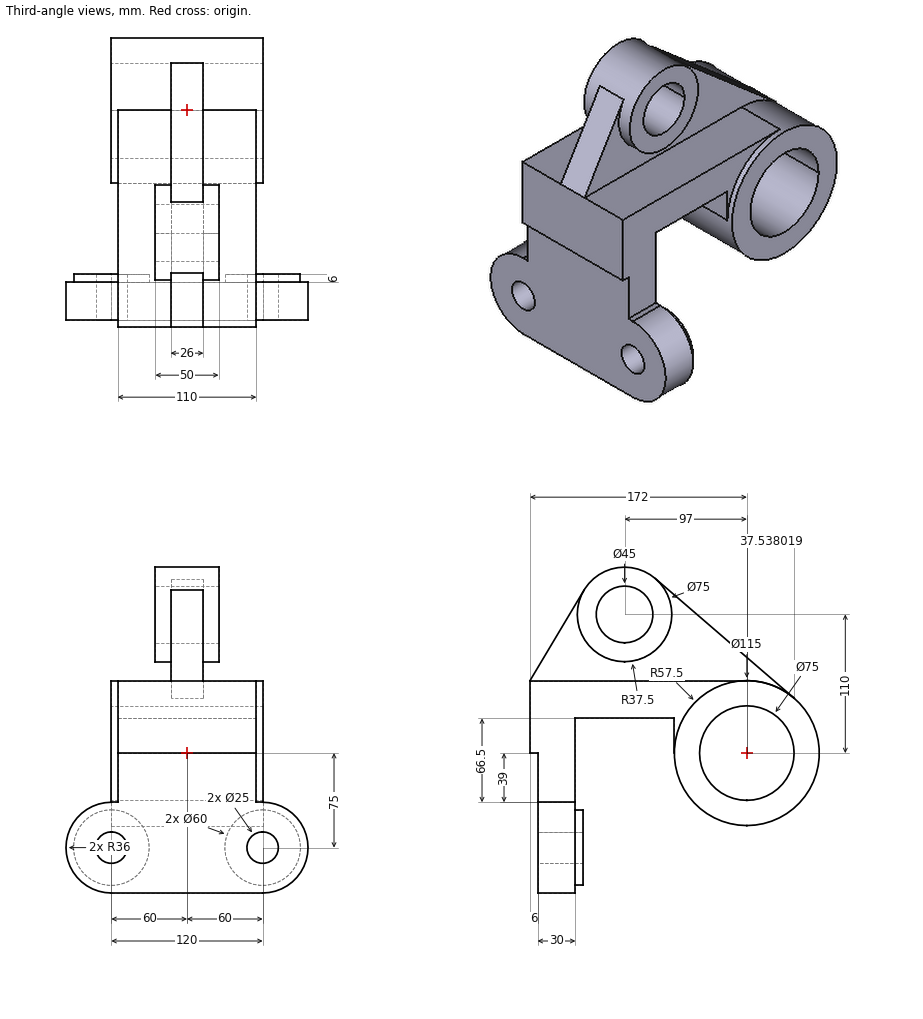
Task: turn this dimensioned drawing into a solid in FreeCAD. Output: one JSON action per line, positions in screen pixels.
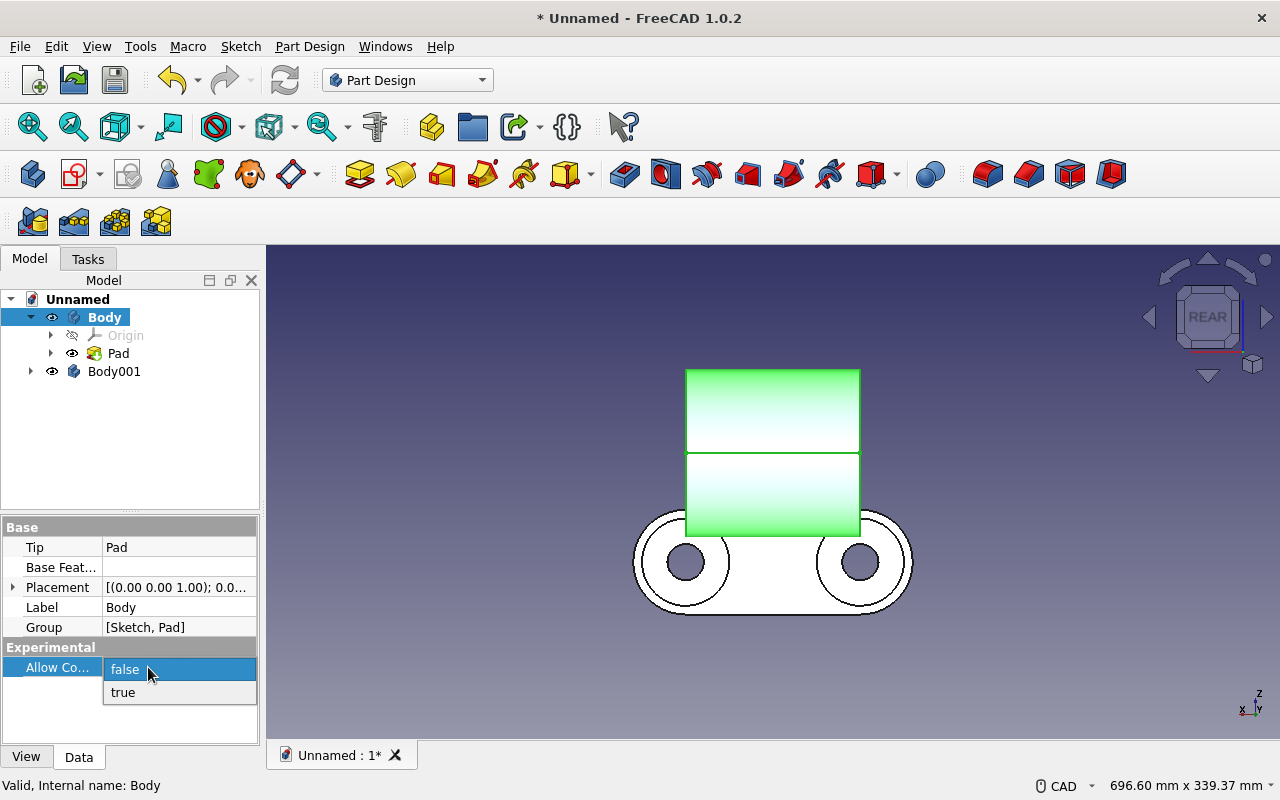
{"action": "left_click", "coordinate": [178, 692]}
{"action": "key", "text": "Return"}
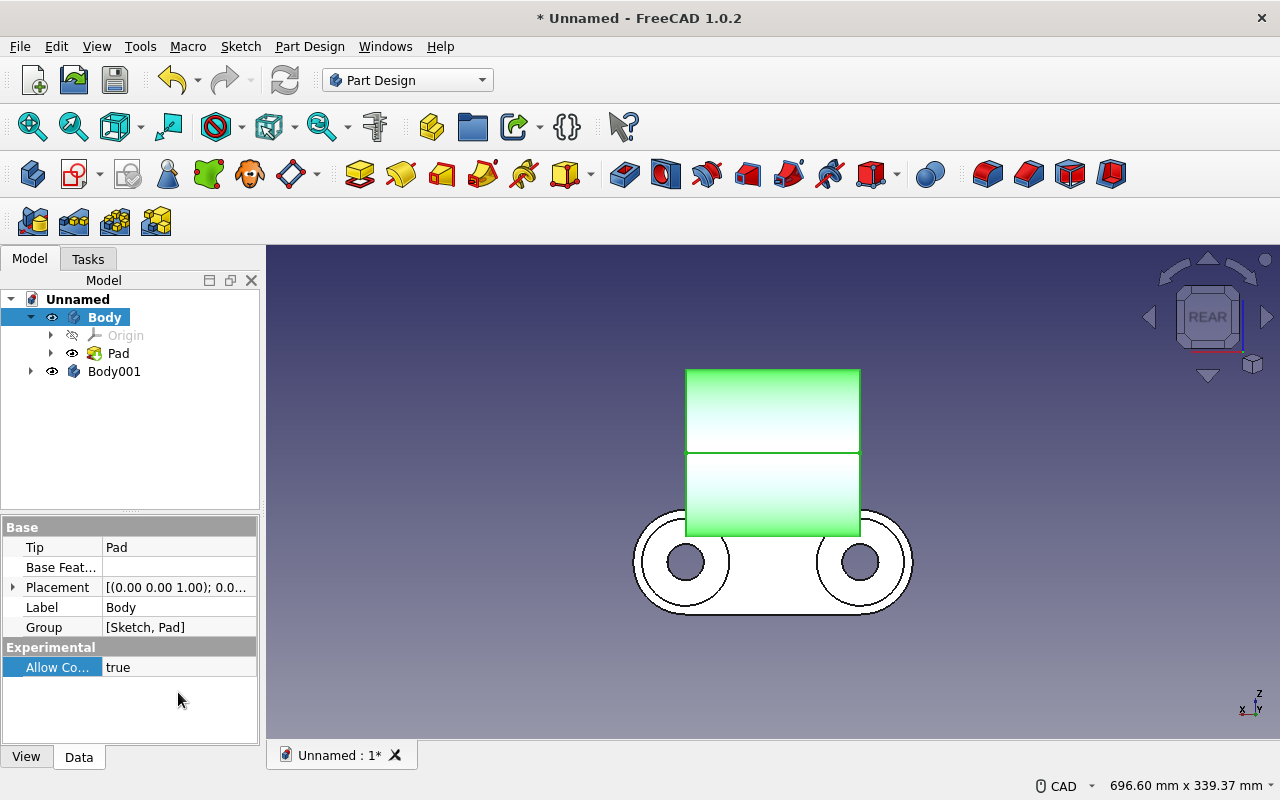
{"action": "left_click", "coordinate": [97, 371]}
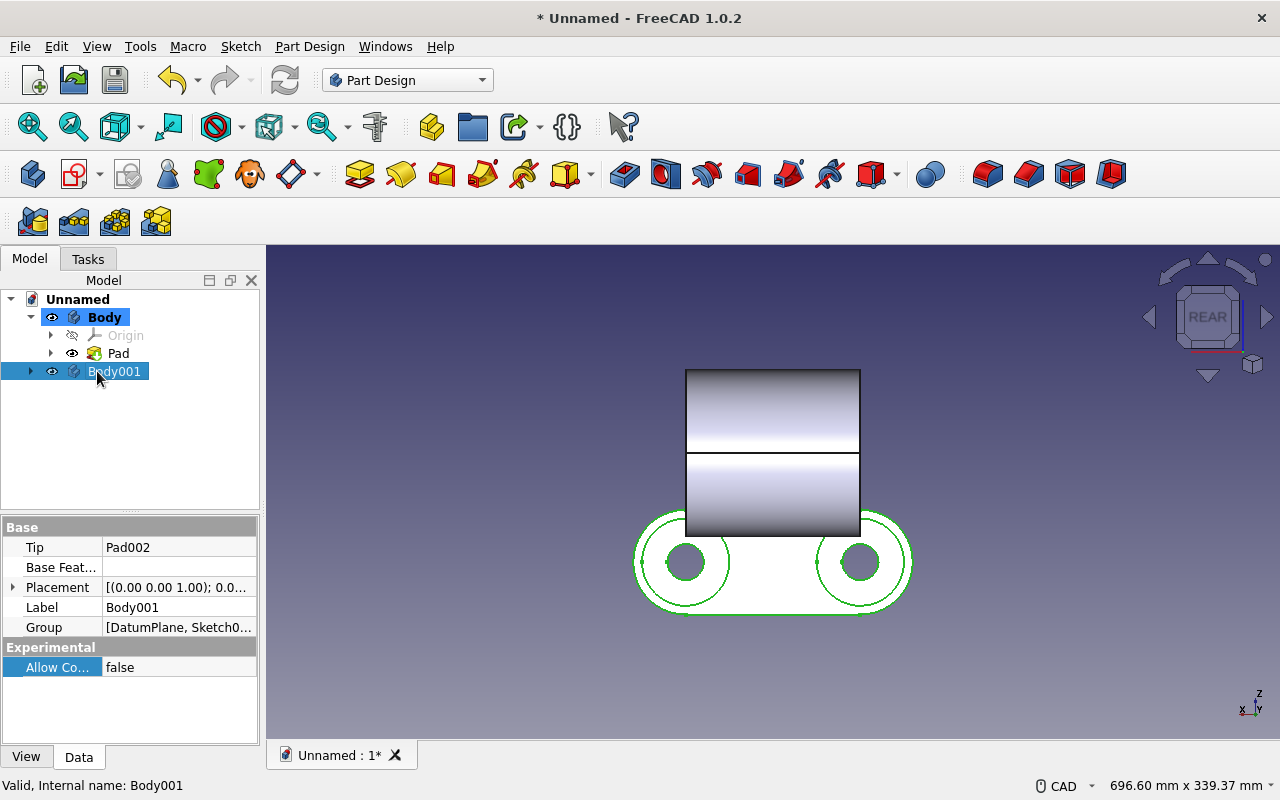
{"action": "left_click", "coordinate": [931, 174]}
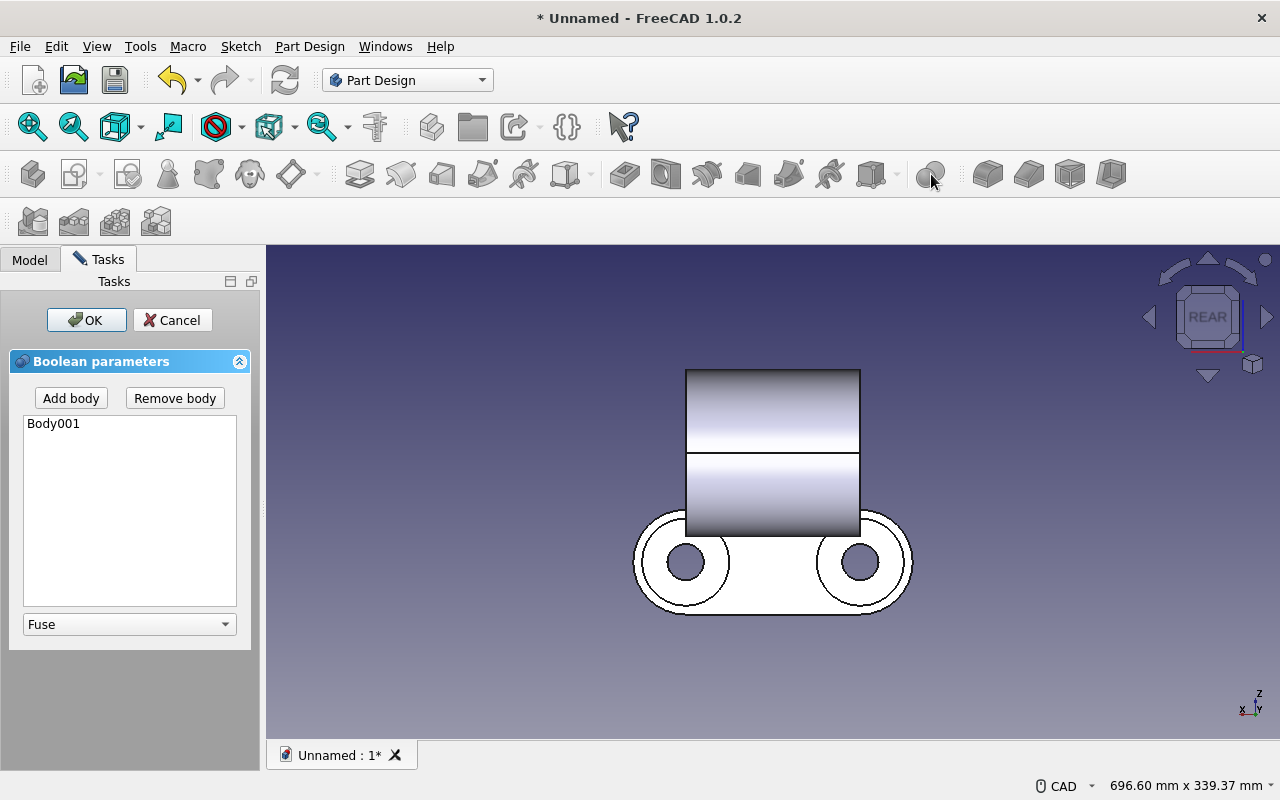
{"action": "left_click", "coordinate": [87, 320]}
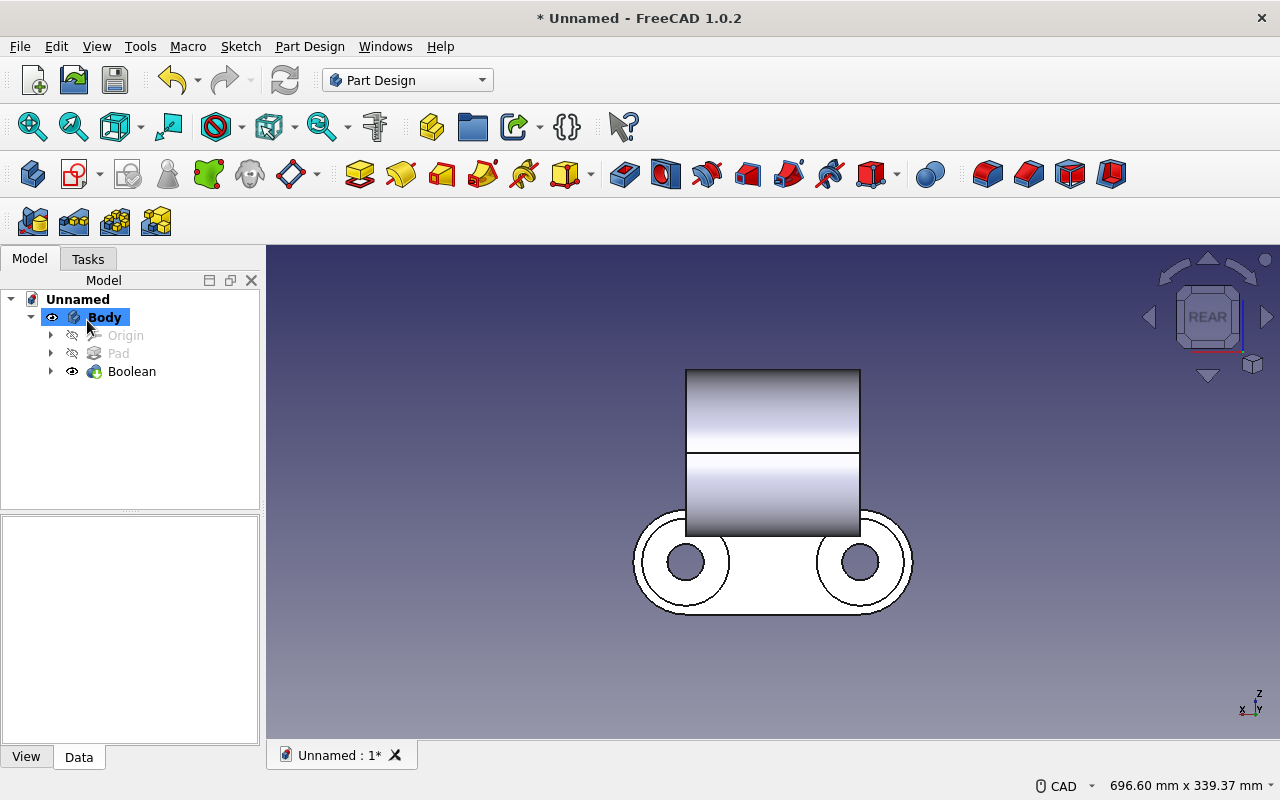
{"action": "left_click", "coordinate": [74, 174]}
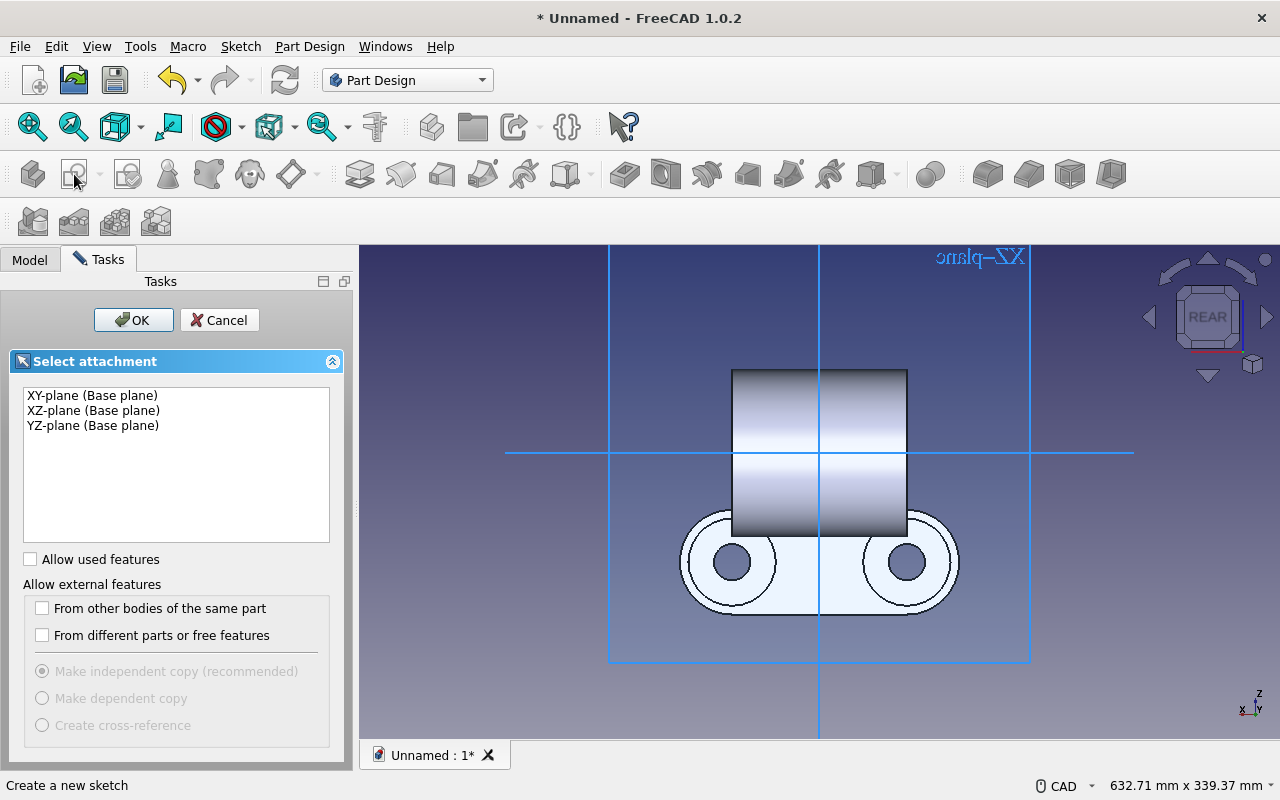
{"action": "left_click", "coordinate": [84, 426]}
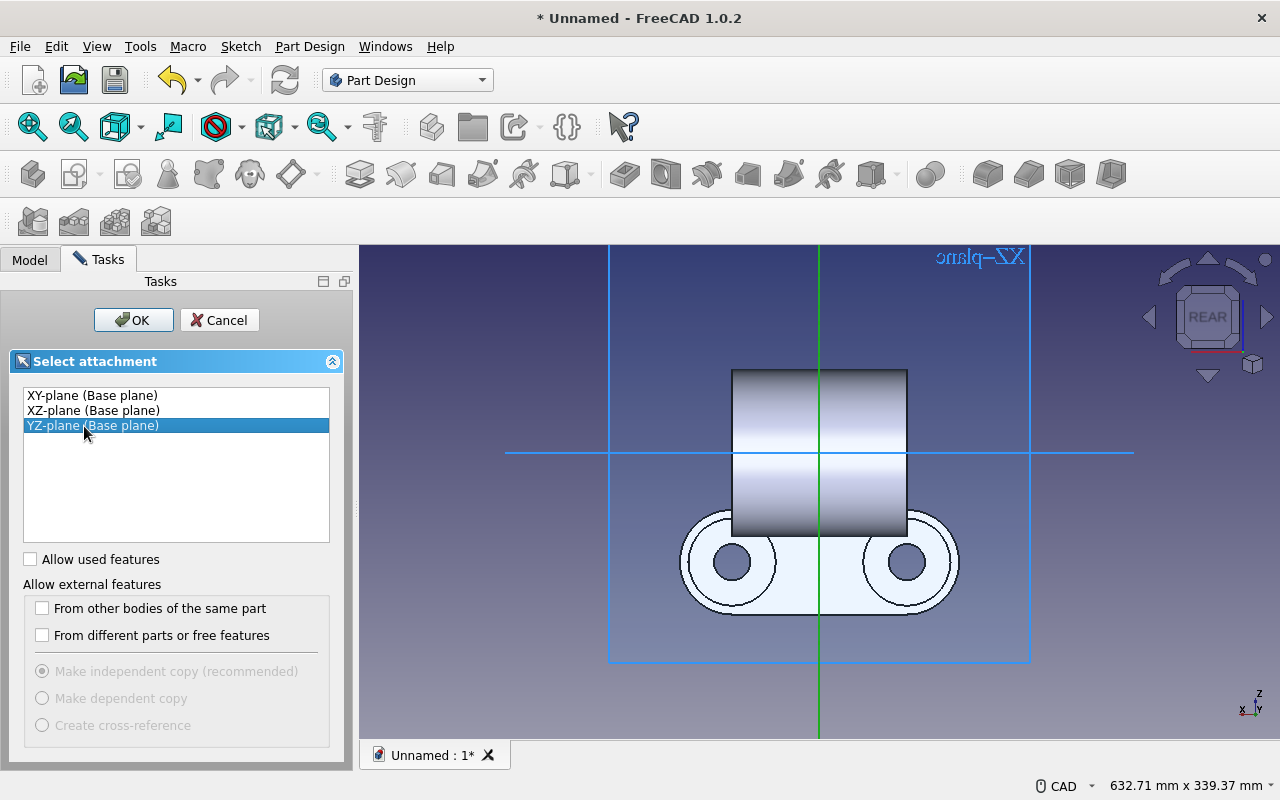
{"action": "left_click", "coordinate": [134, 320]}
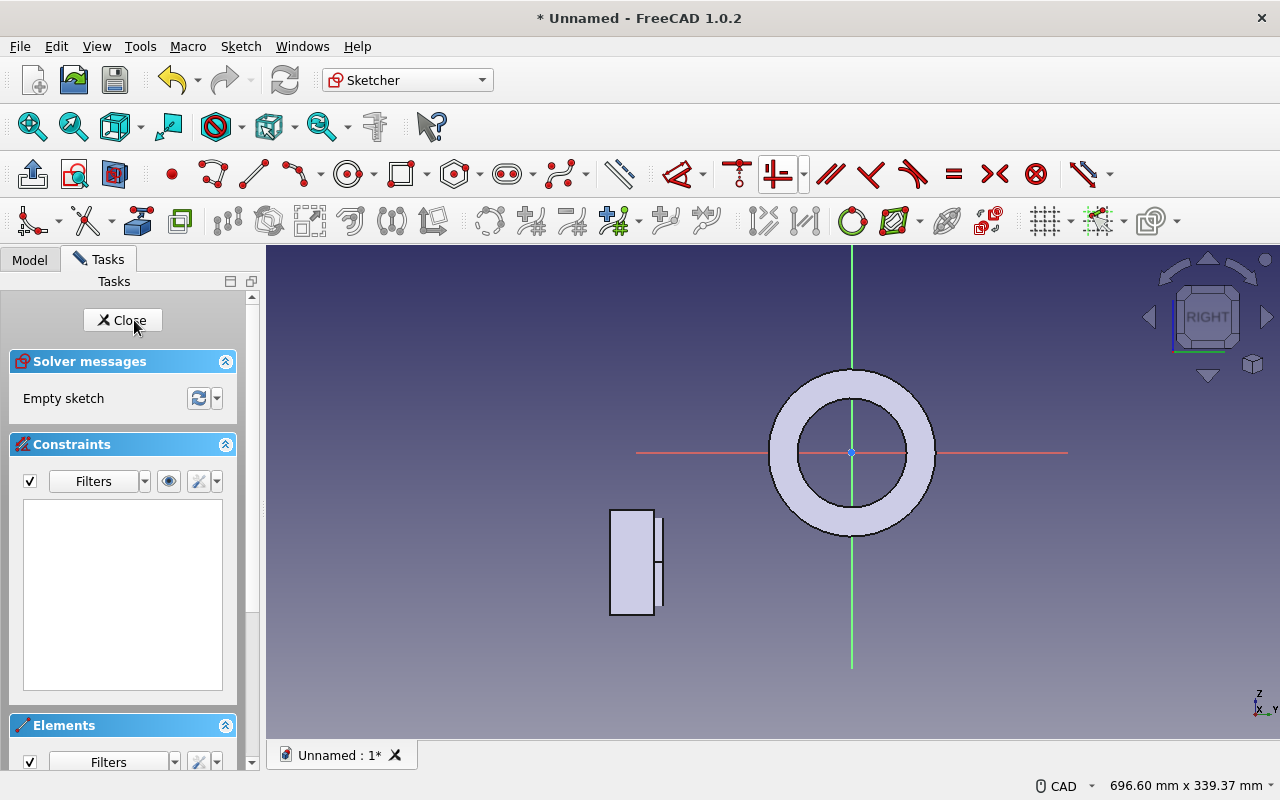
{"action": "key", "text": "q s"}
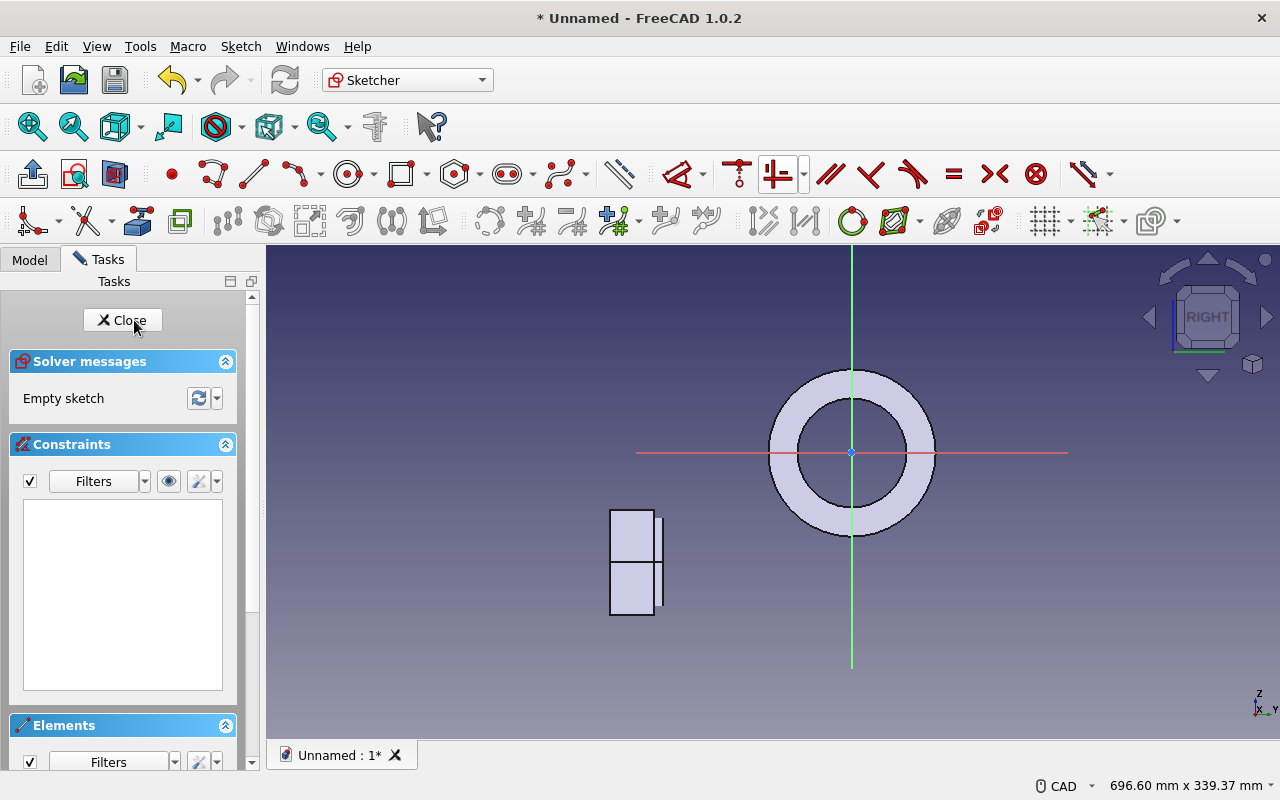
{"action": "scroll", "coordinate": [745, 397], "scroll_direction": "up", "scroll_amount": 4}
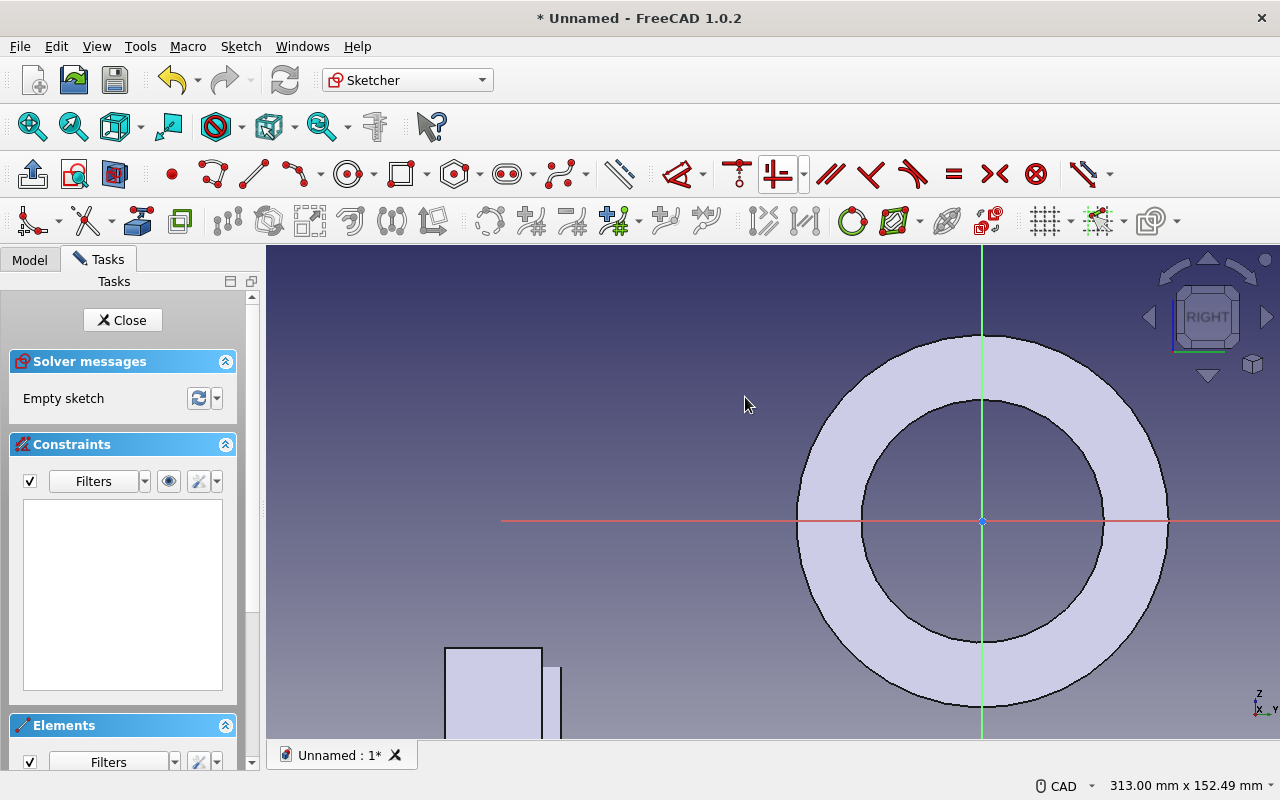
{"action": "key", "text": "g m"}